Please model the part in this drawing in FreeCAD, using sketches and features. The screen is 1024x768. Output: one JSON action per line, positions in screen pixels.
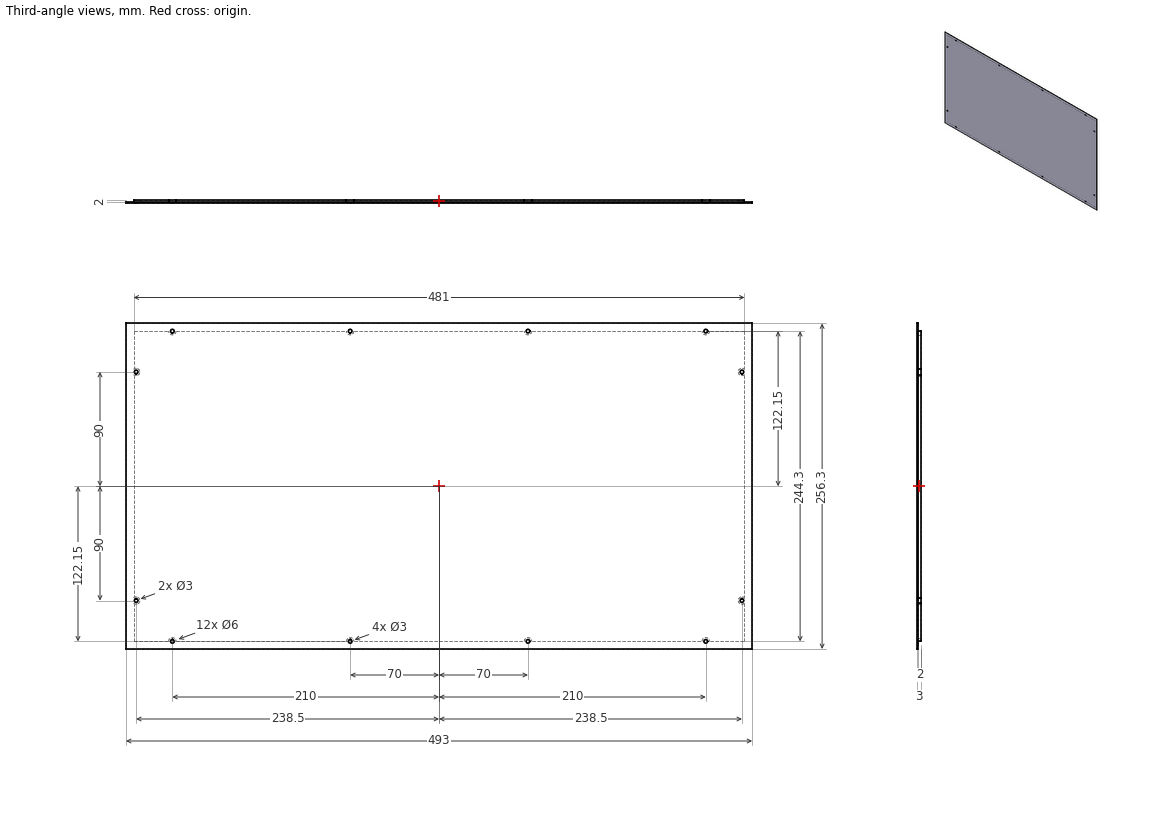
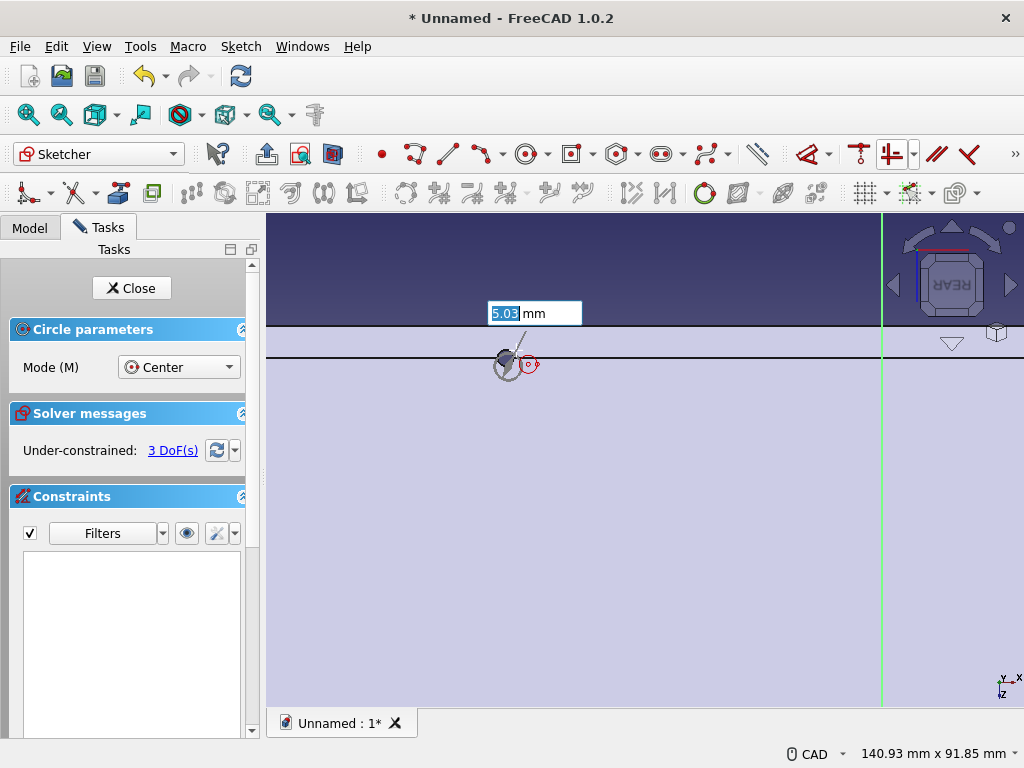
{"action": "left_click", "coordinate": [517, 347]}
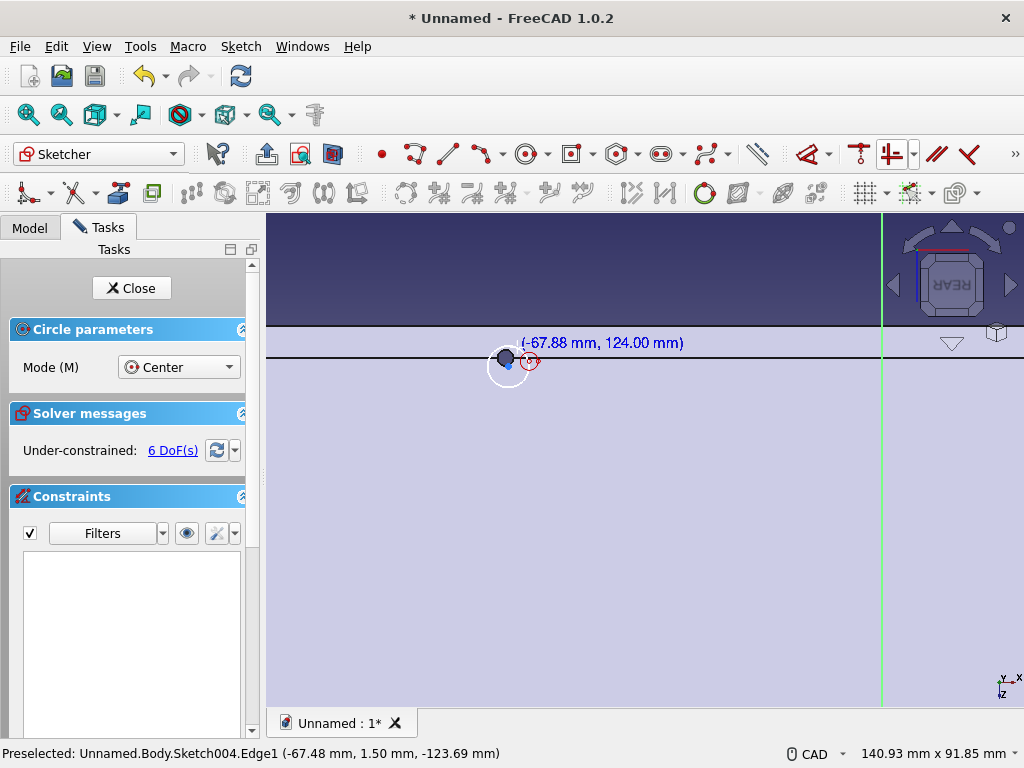
{"action": "scroll", "coordinate": [516, 350], "scroll_direction": "down", "scroll_amount": 9}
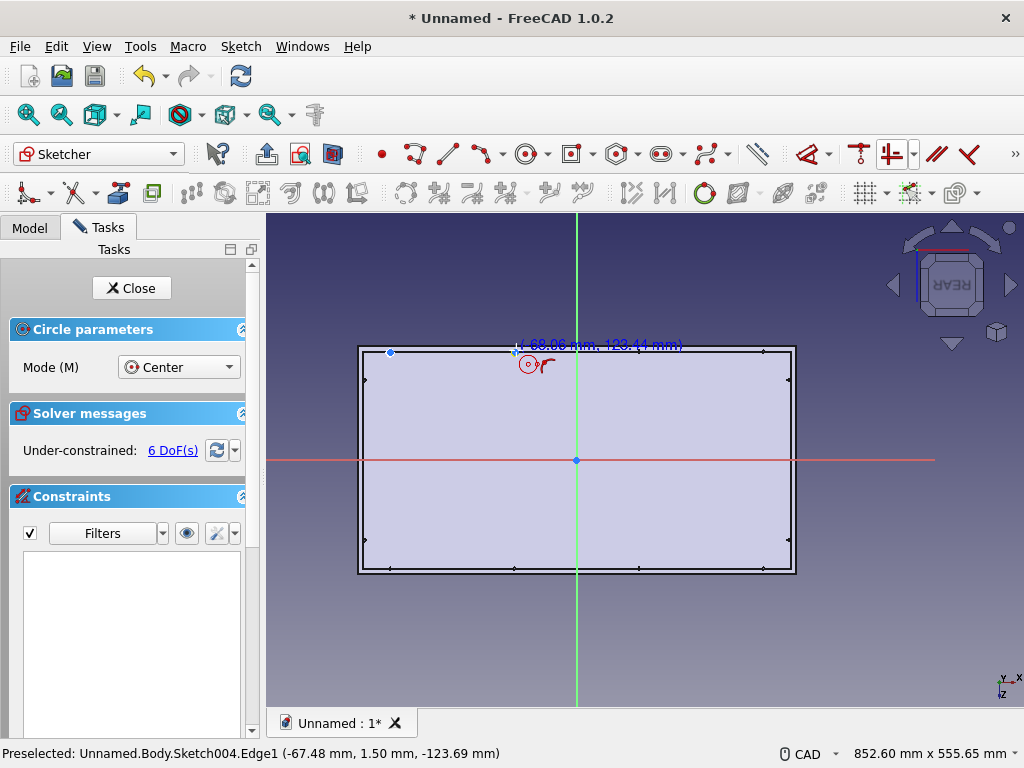
{"action": "scroll", "coordinate": [639, 352], "scroll_direction": "up", "scroll_amount": 11}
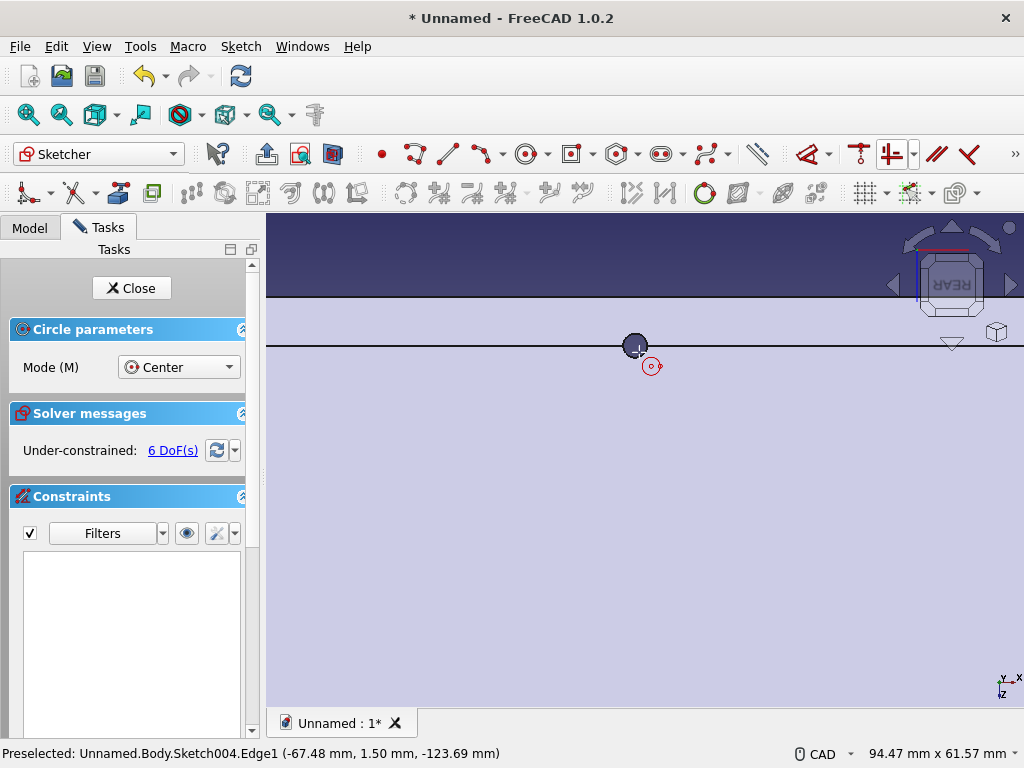
{"action": "scroll", "coordinate": [639, 352], "scroll_direction": "down", "scroll_amount": 11}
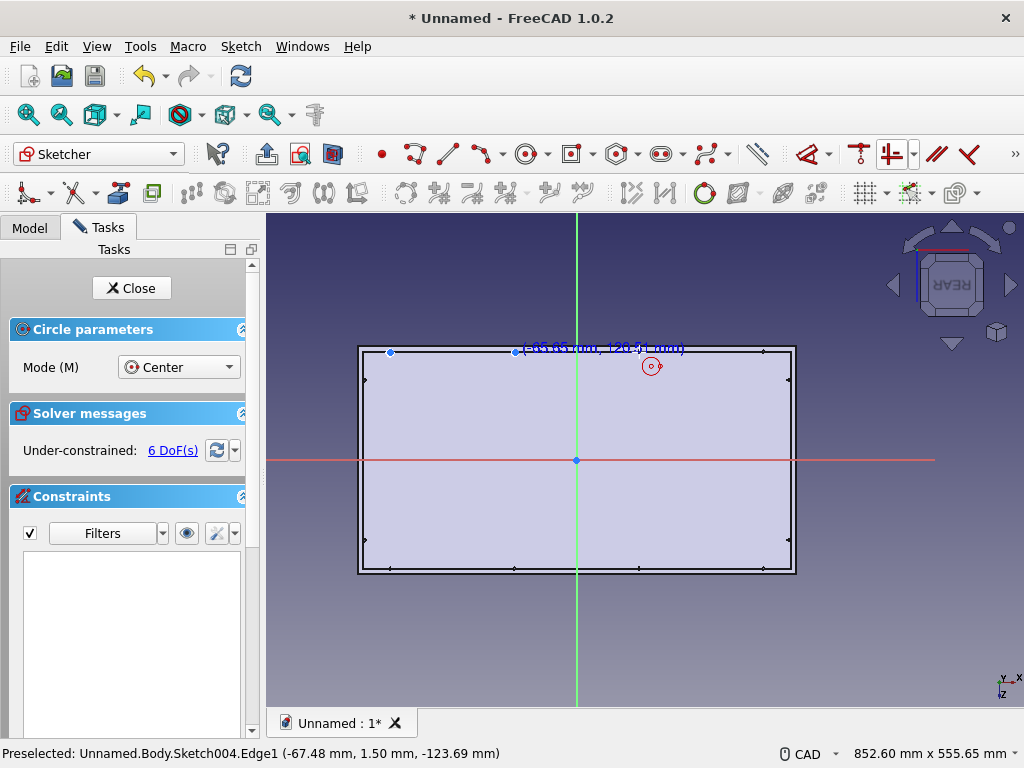
{"action": "left_click", "coordinate": [639, 352]}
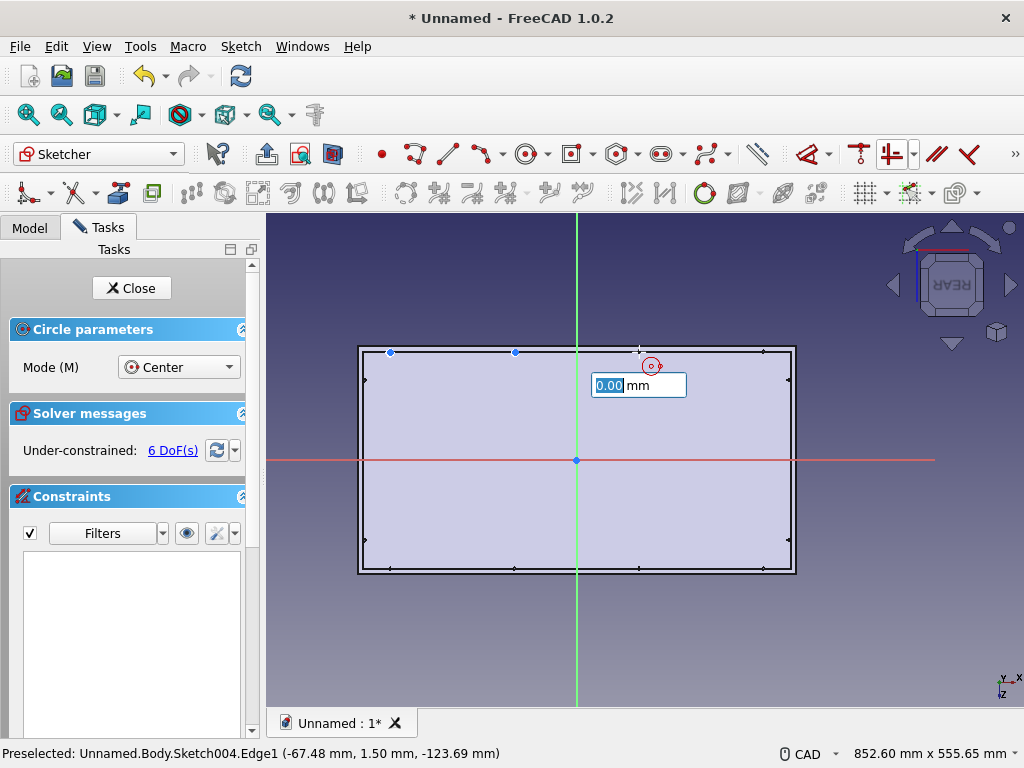
{"action": "scroll", "coordinate": [641, 350], "scroll_direction": "up", "scroll_amount": 9}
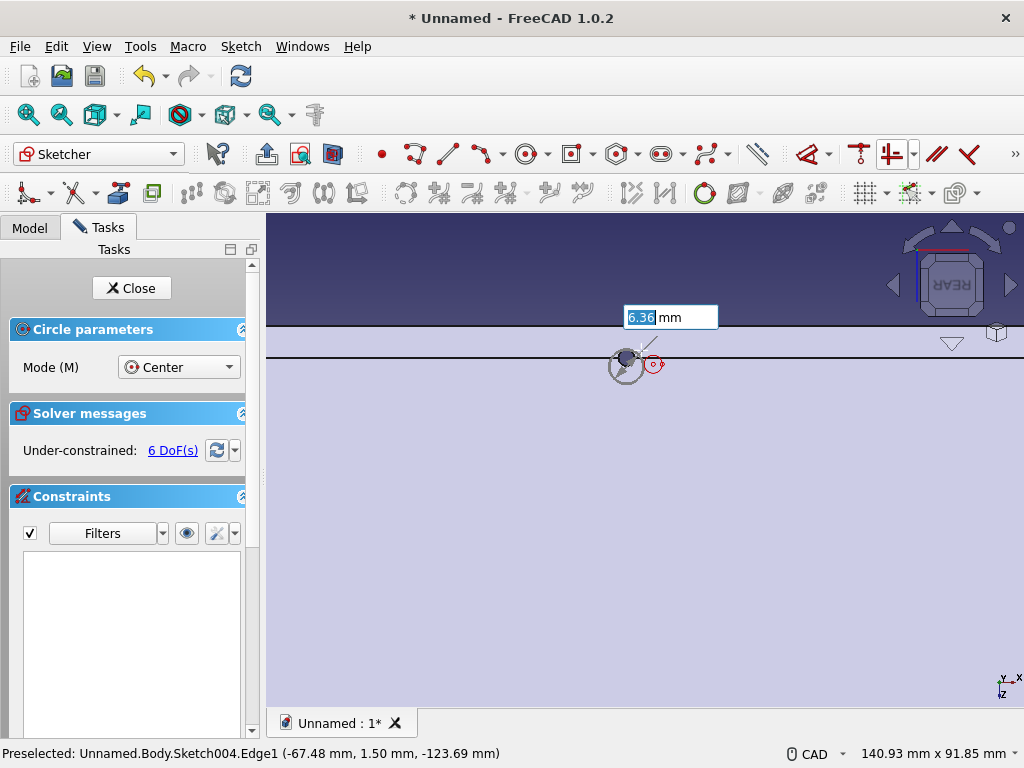
{"action": "left_click", "coordinate": [638, 347]}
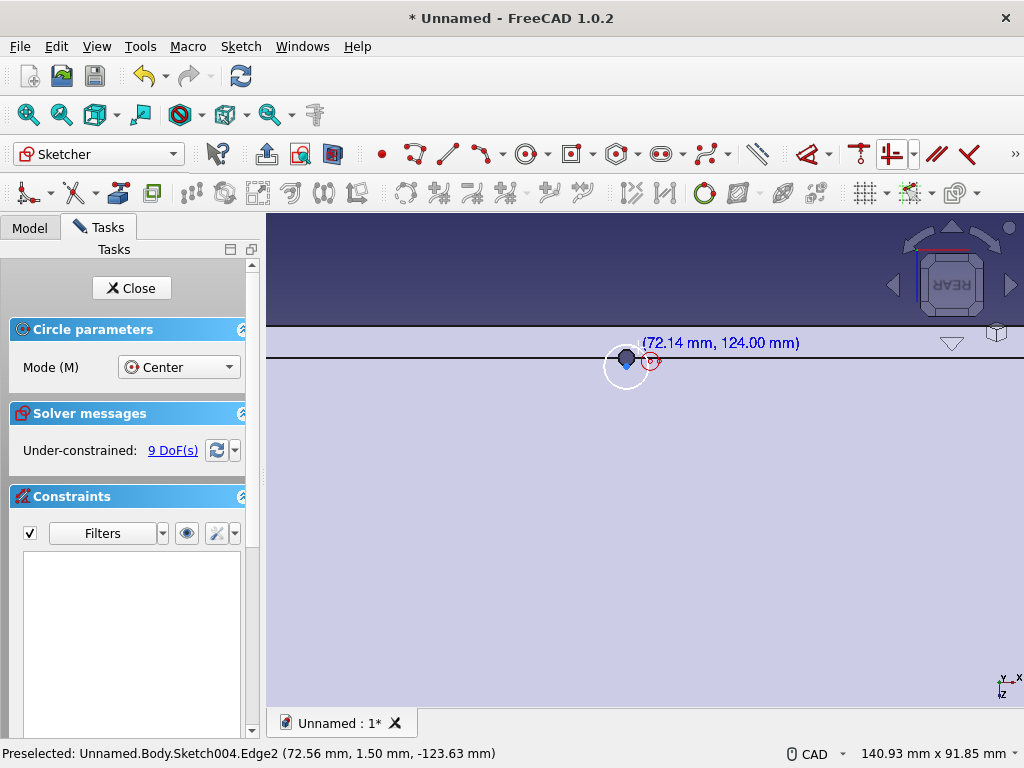
{"action": "scroll", "coordinate": [641, 350], "scroll_direction": "down", "scroll_amount": 9}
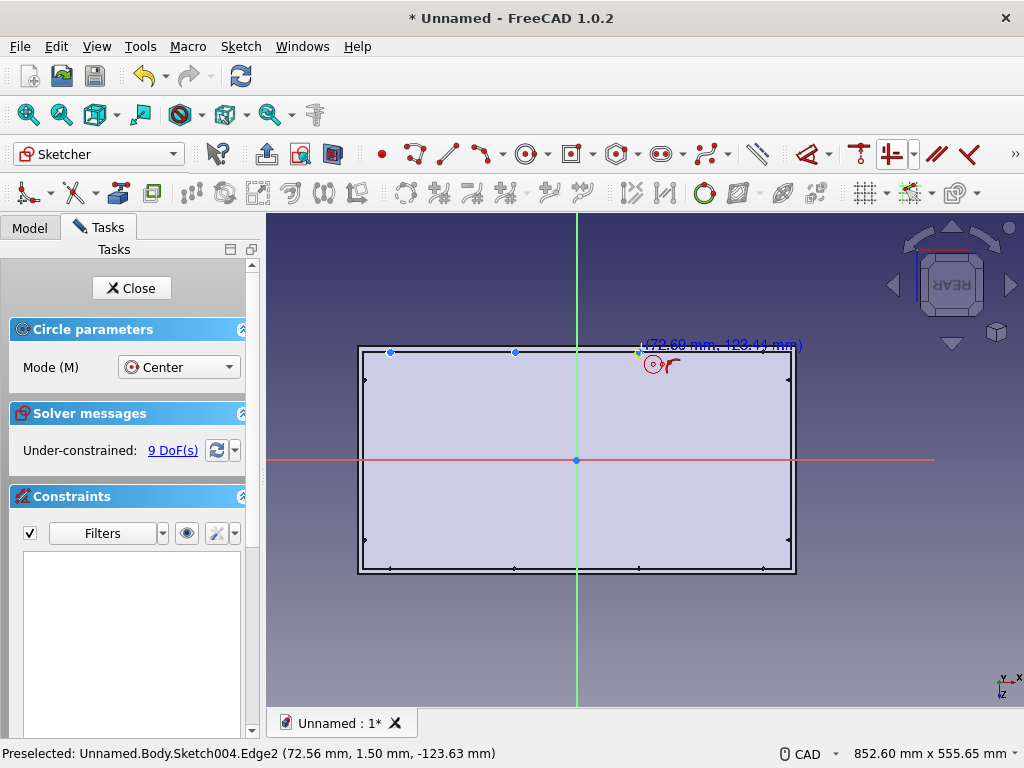
{"action": "scroll", "coordinate": [763, 352], "scroll_direction": "up", "scroll_amount": 11}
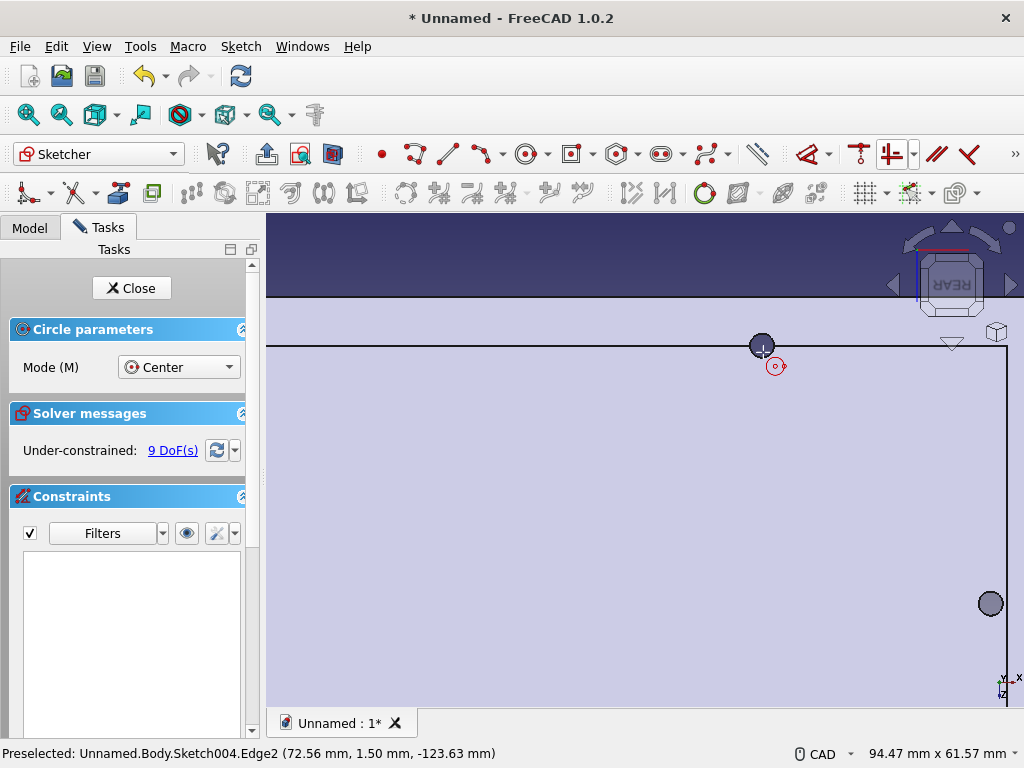
{"action": "scroll", "coordinate": [763, 352], "scroll_direction": "down", "scroll_amount": 11}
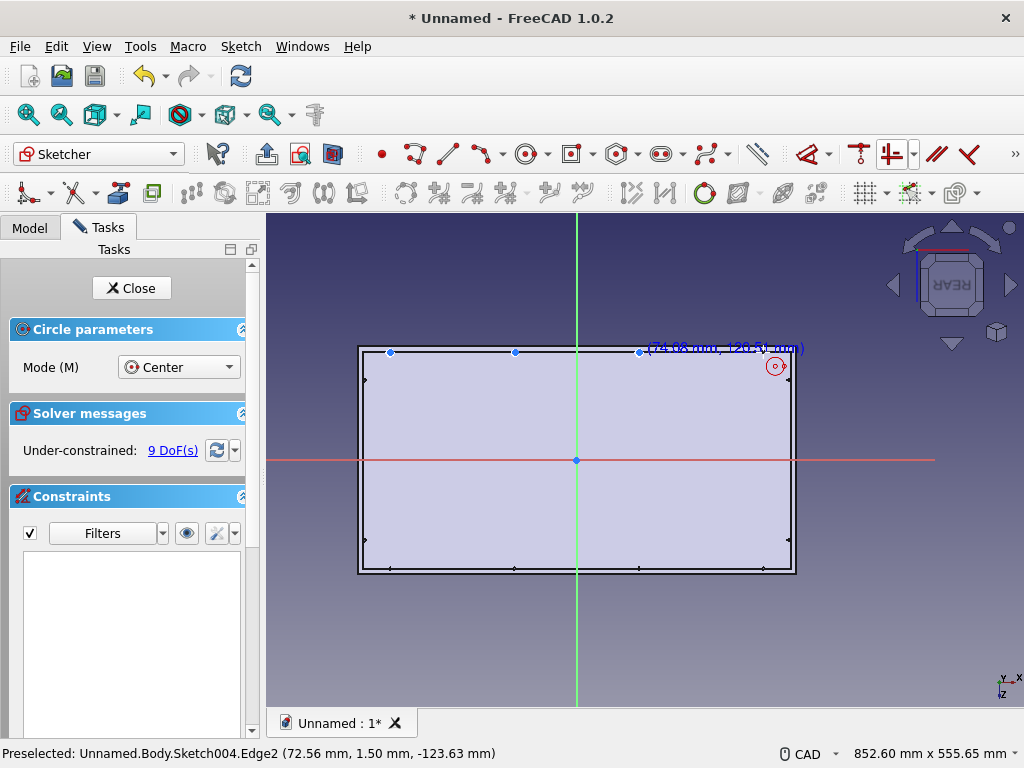
{"action": "left_click", "coordinate": [763, 352]}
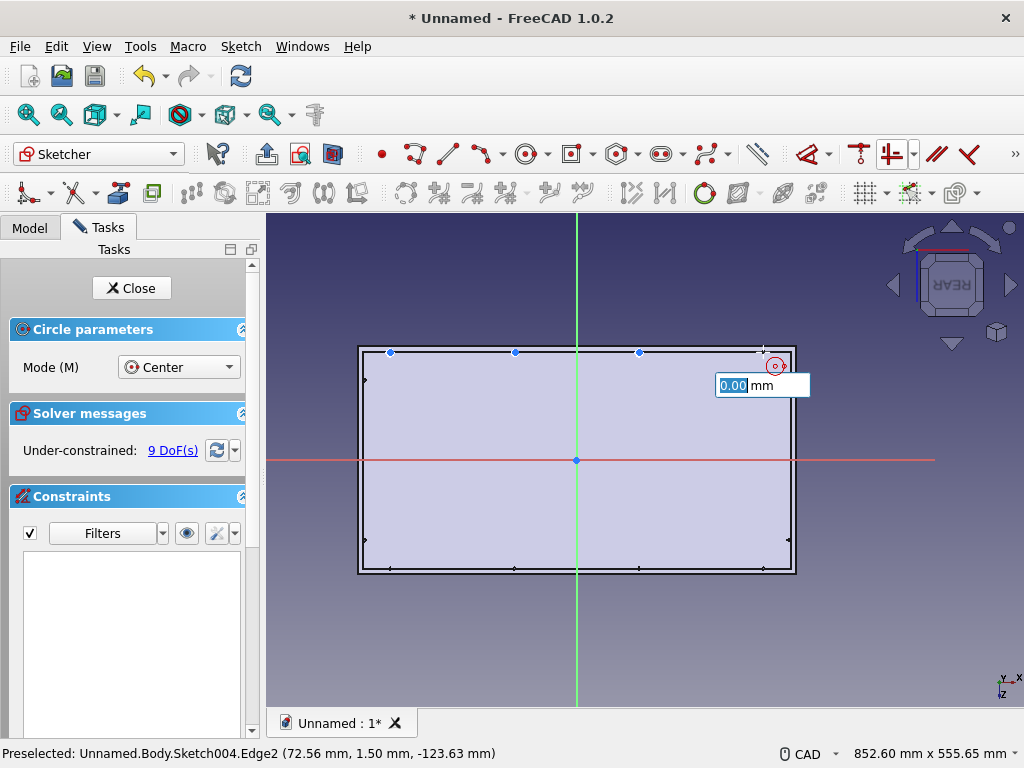
{"action": "scroll", "coordinate": [765, 350], "scroll_direction": "up", "scroll_amount": 9}